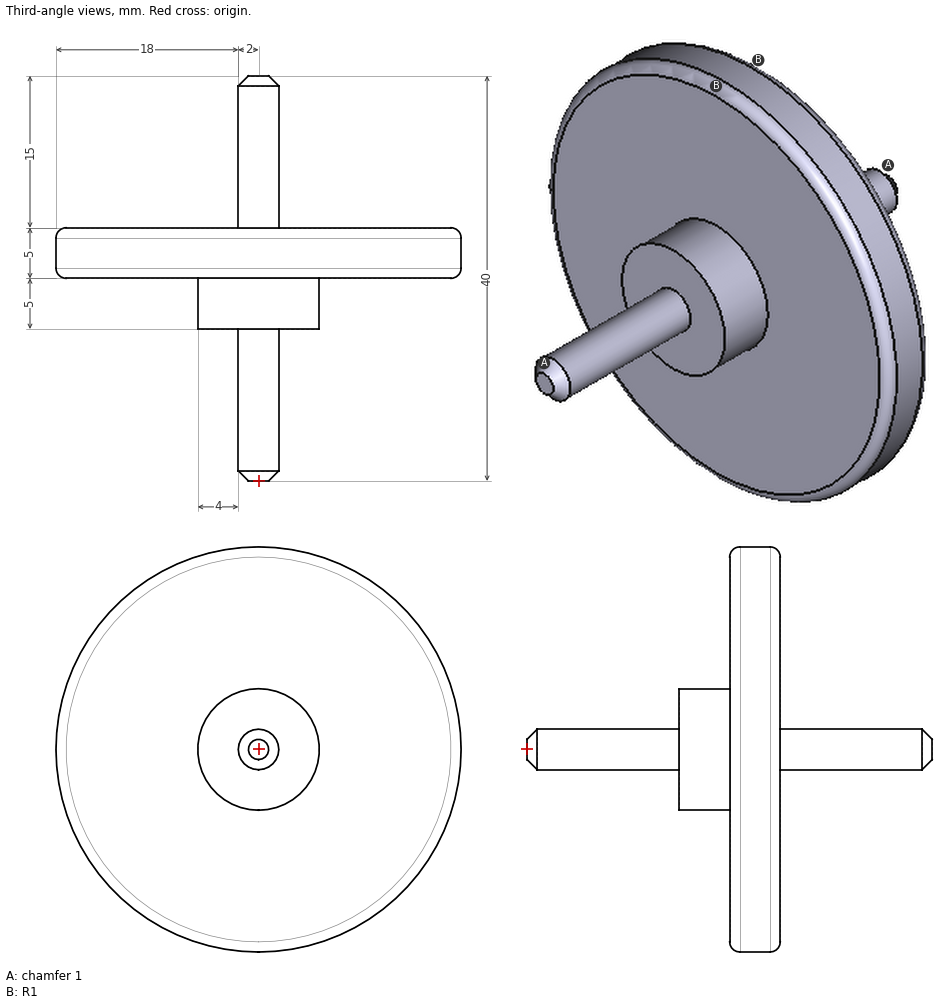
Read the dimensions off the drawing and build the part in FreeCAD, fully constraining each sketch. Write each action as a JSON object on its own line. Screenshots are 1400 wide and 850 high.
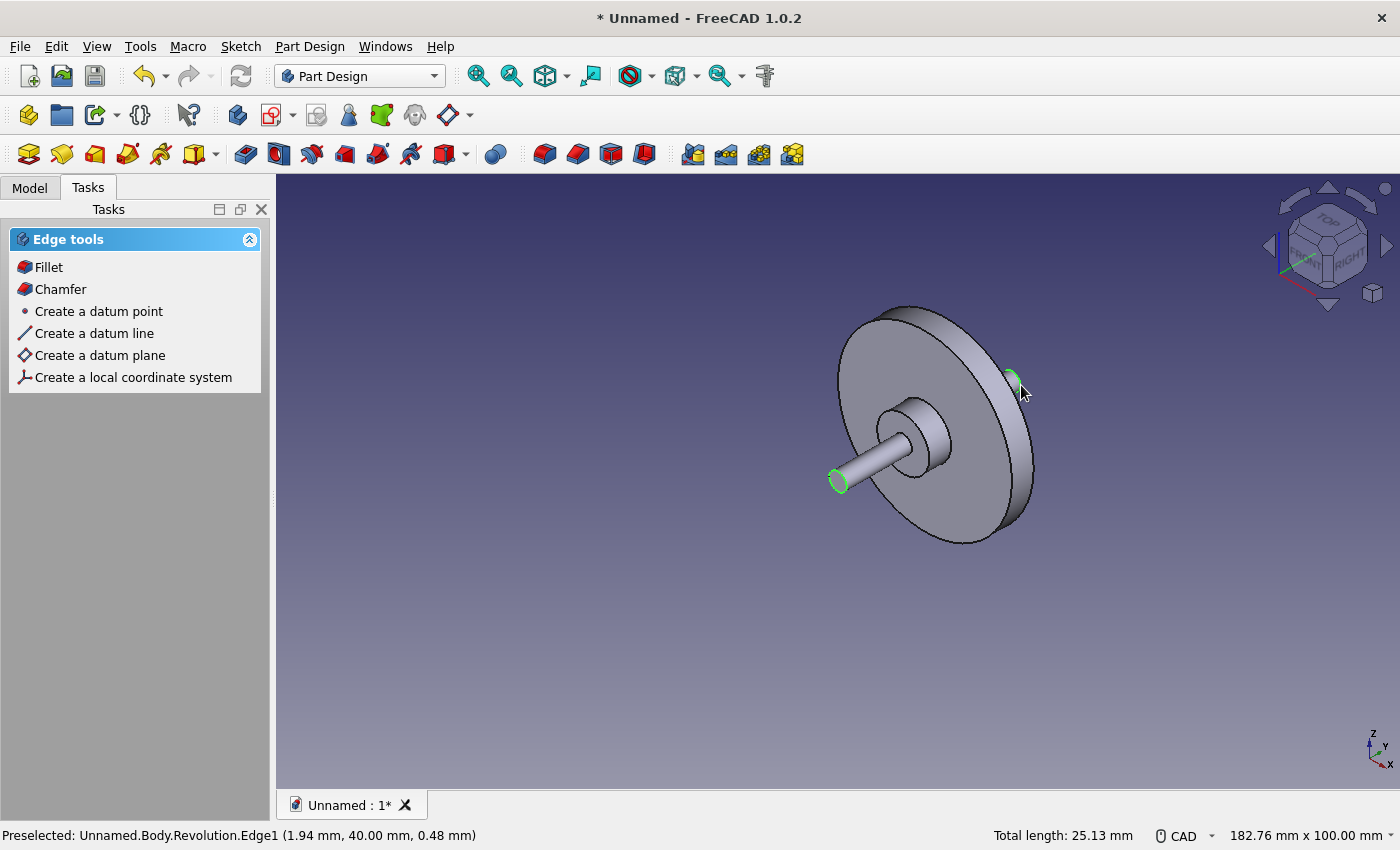
{"action": "left_click", "coordinate": [578, 154]}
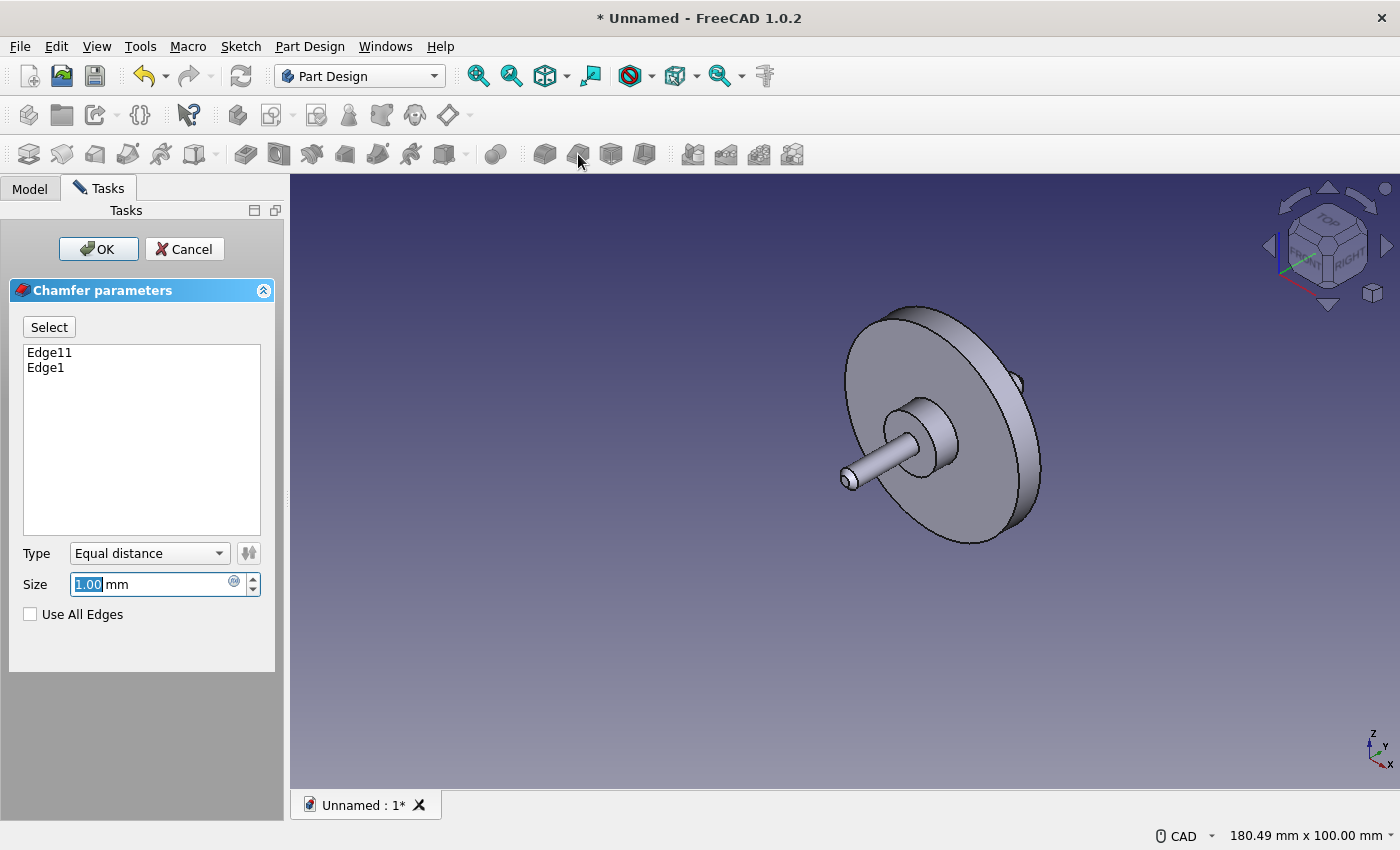
{"action": "type", "text": "1"}
{"action": "key", "text": "Tab"}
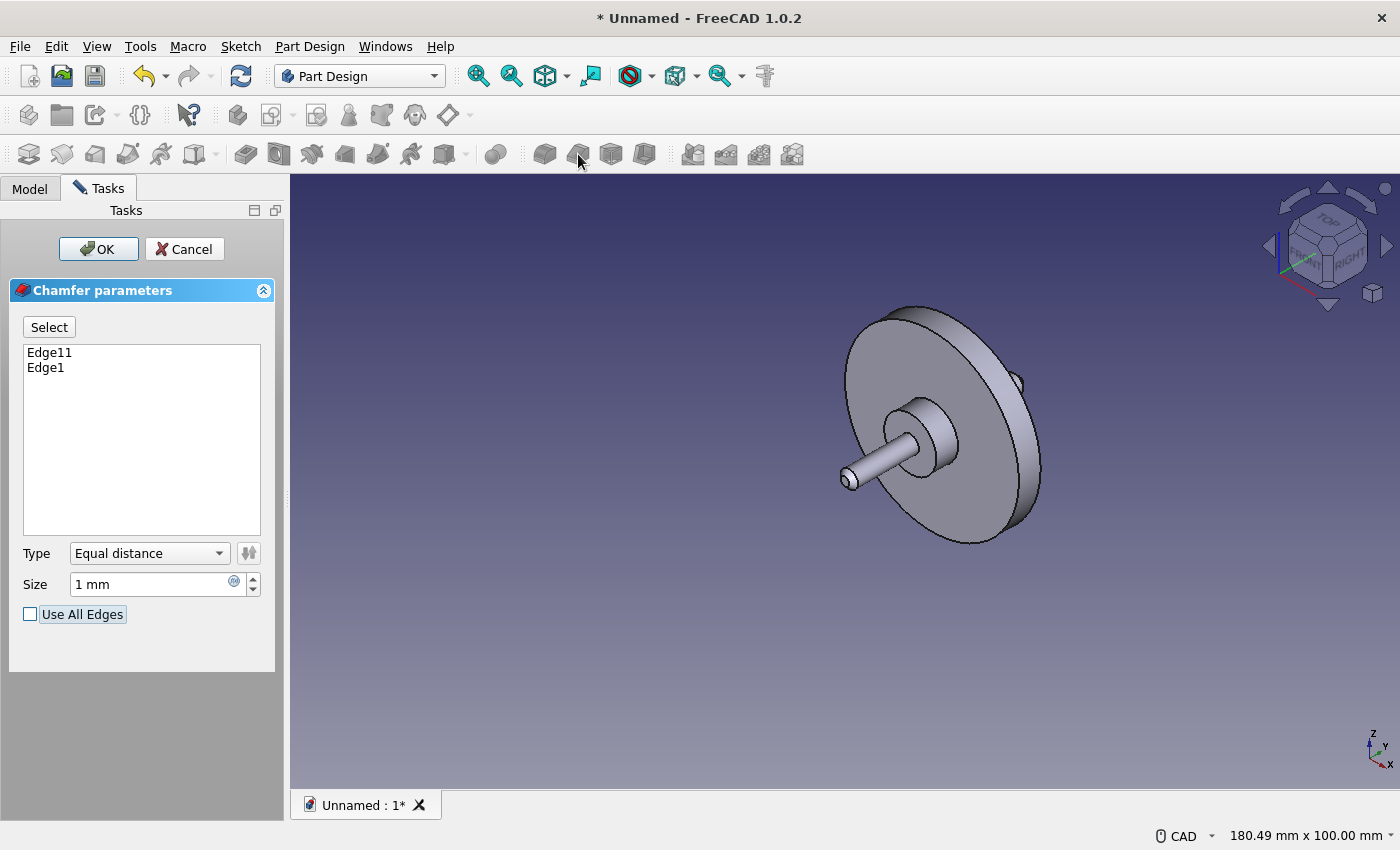
{"action": "left_click", "coordinate": [99, 249]}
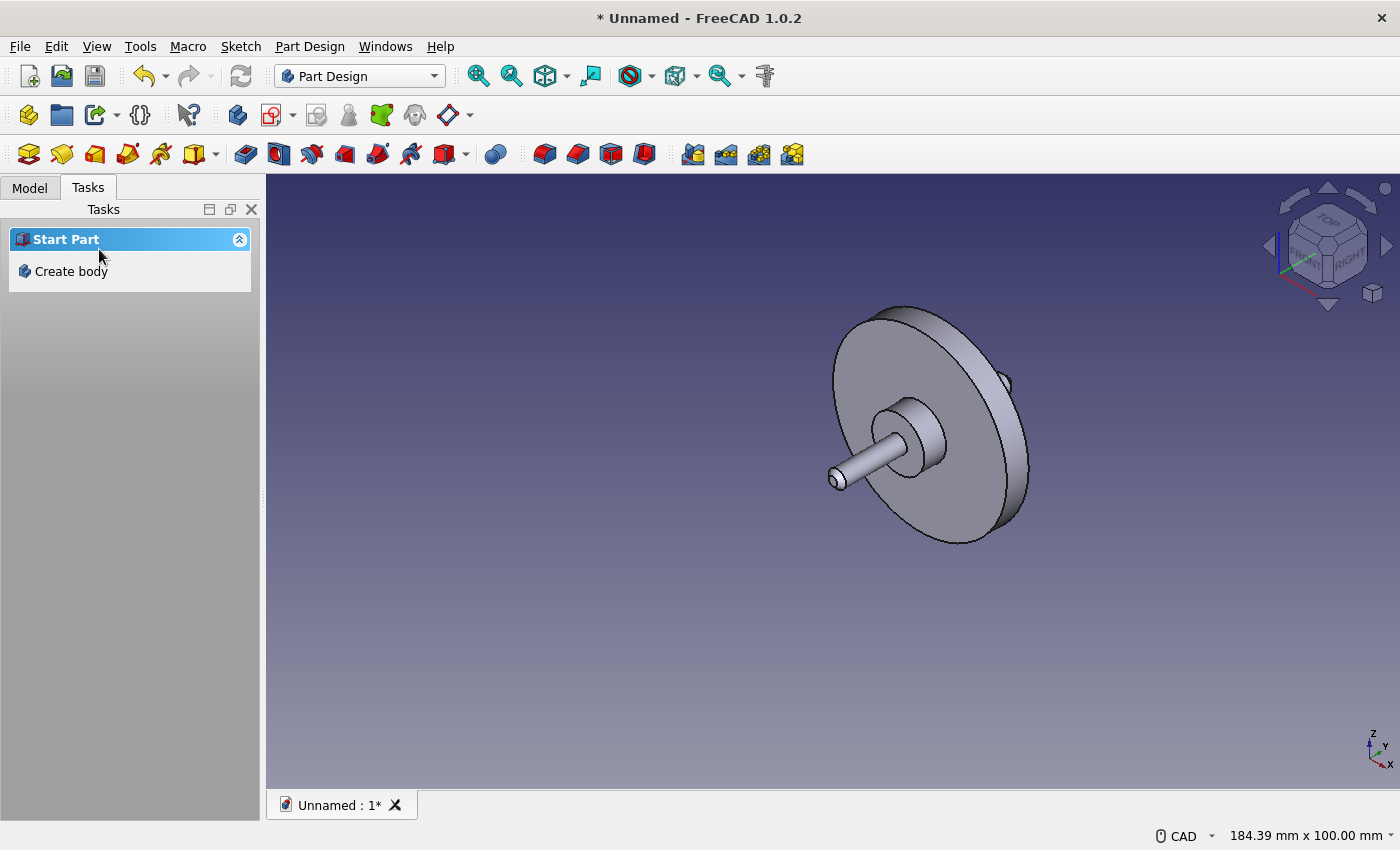
{"action": "left_click", "coordinate": [1007, 480]}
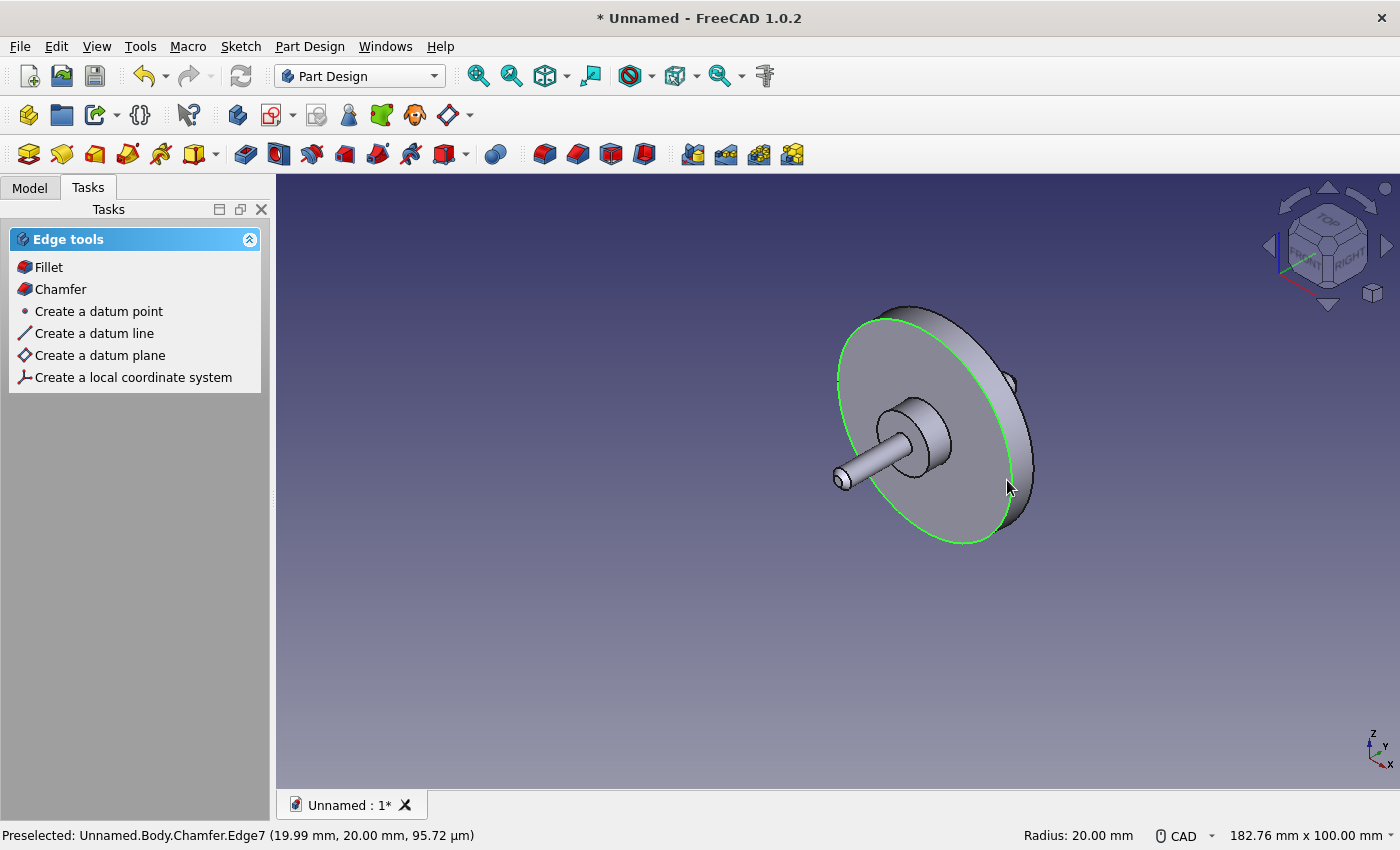
{"action": "key", "text": "2"}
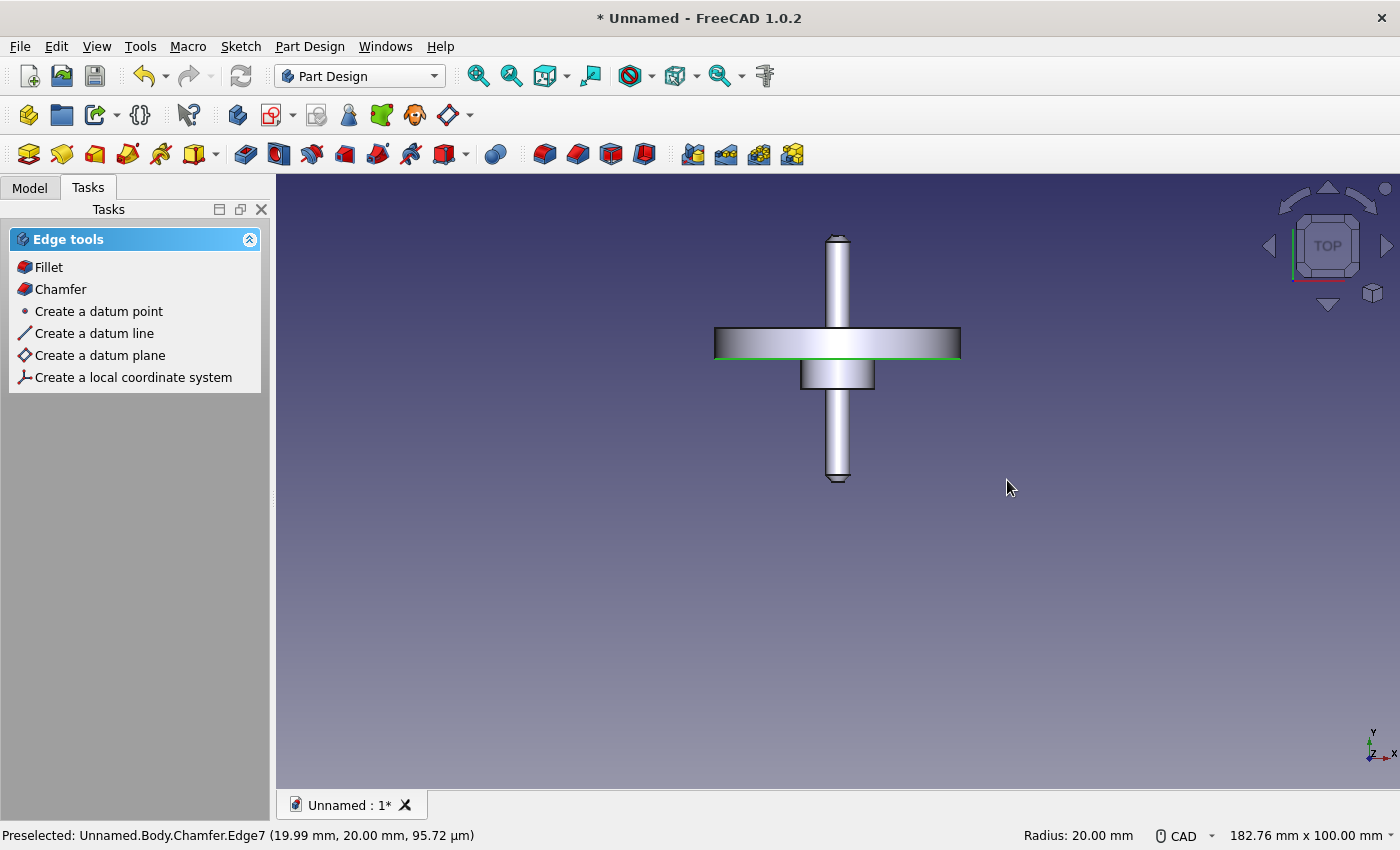
{"action": "left_click", "coordinate": [479, 76]}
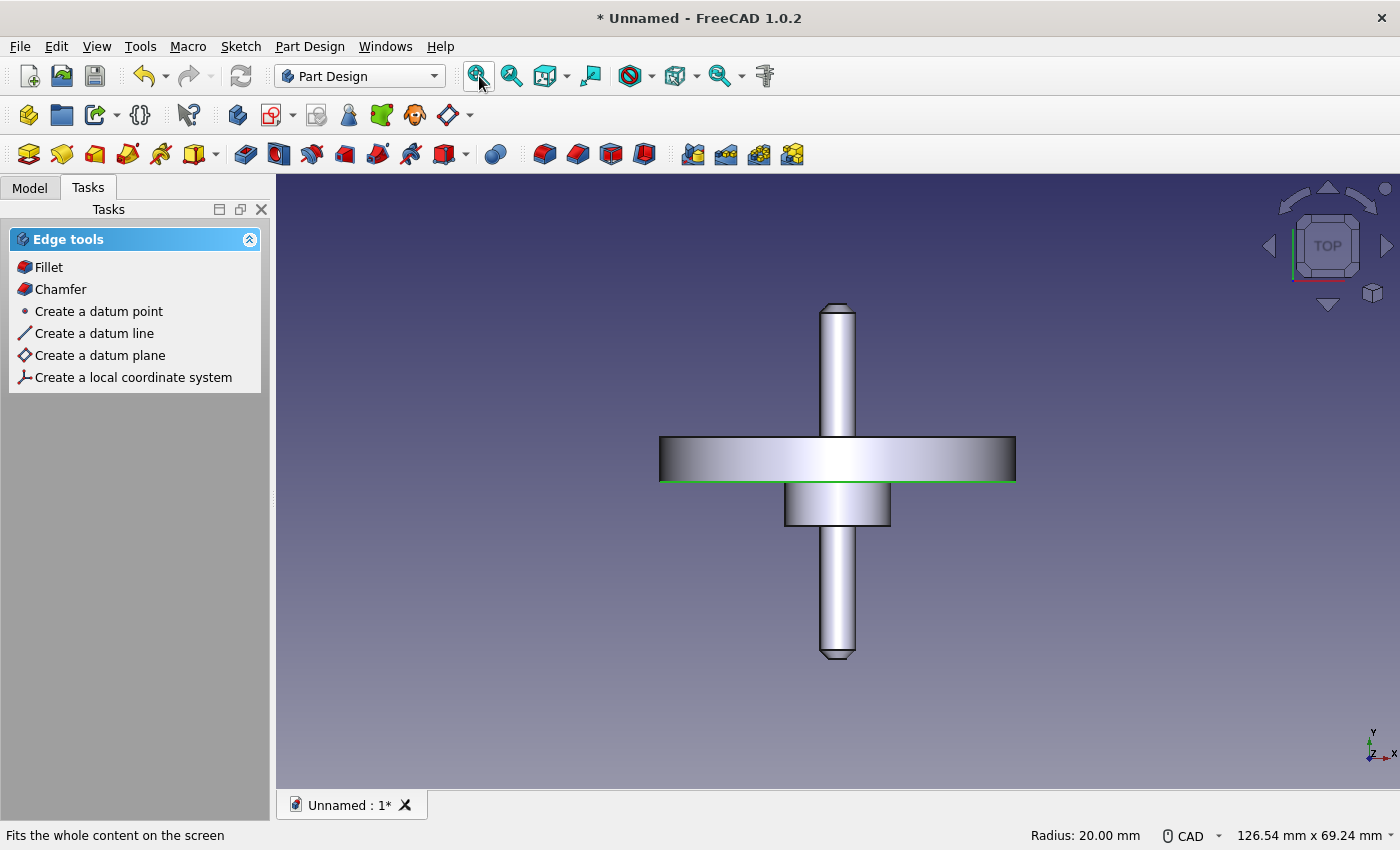
{"action": "left_click", "coordinate": [982, 436], "text": "ctrl"}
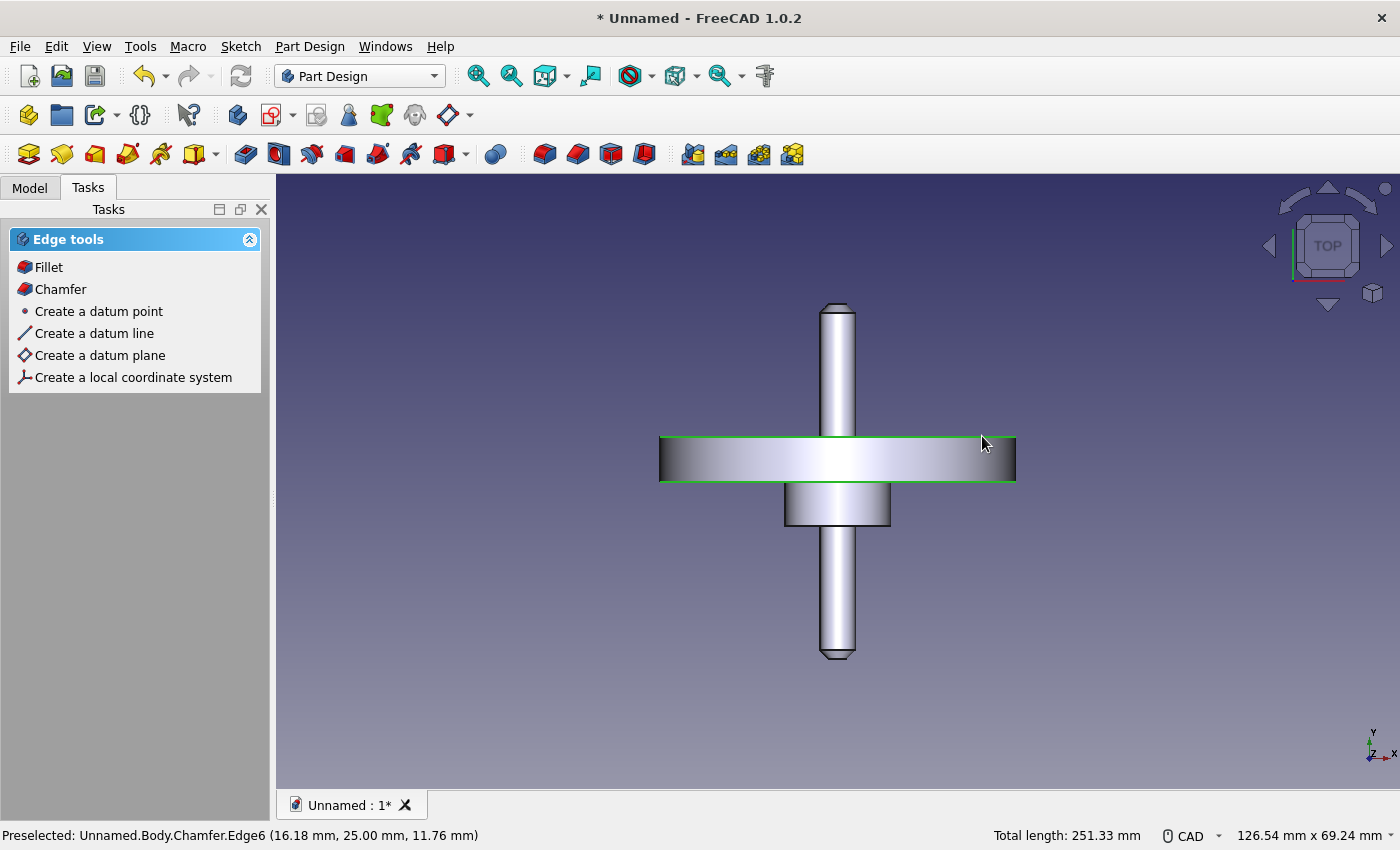
{"action": "left_click", "coordinate": [545, 154]}